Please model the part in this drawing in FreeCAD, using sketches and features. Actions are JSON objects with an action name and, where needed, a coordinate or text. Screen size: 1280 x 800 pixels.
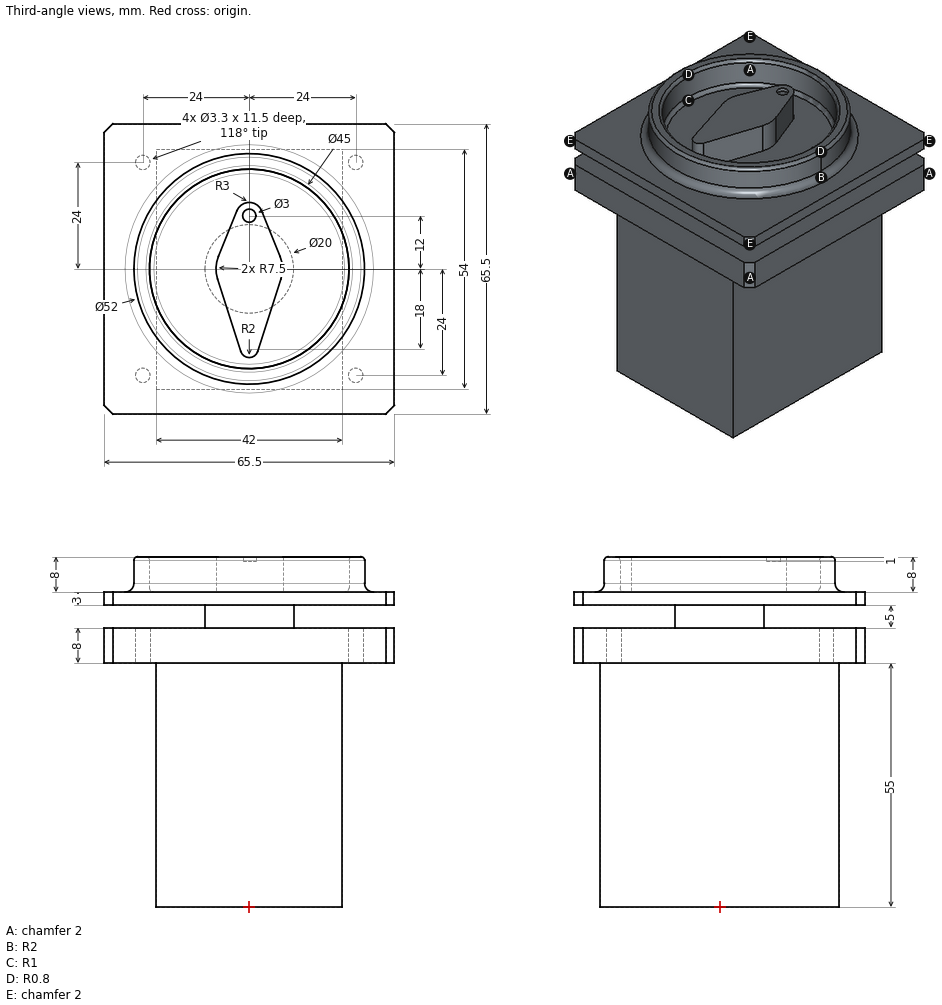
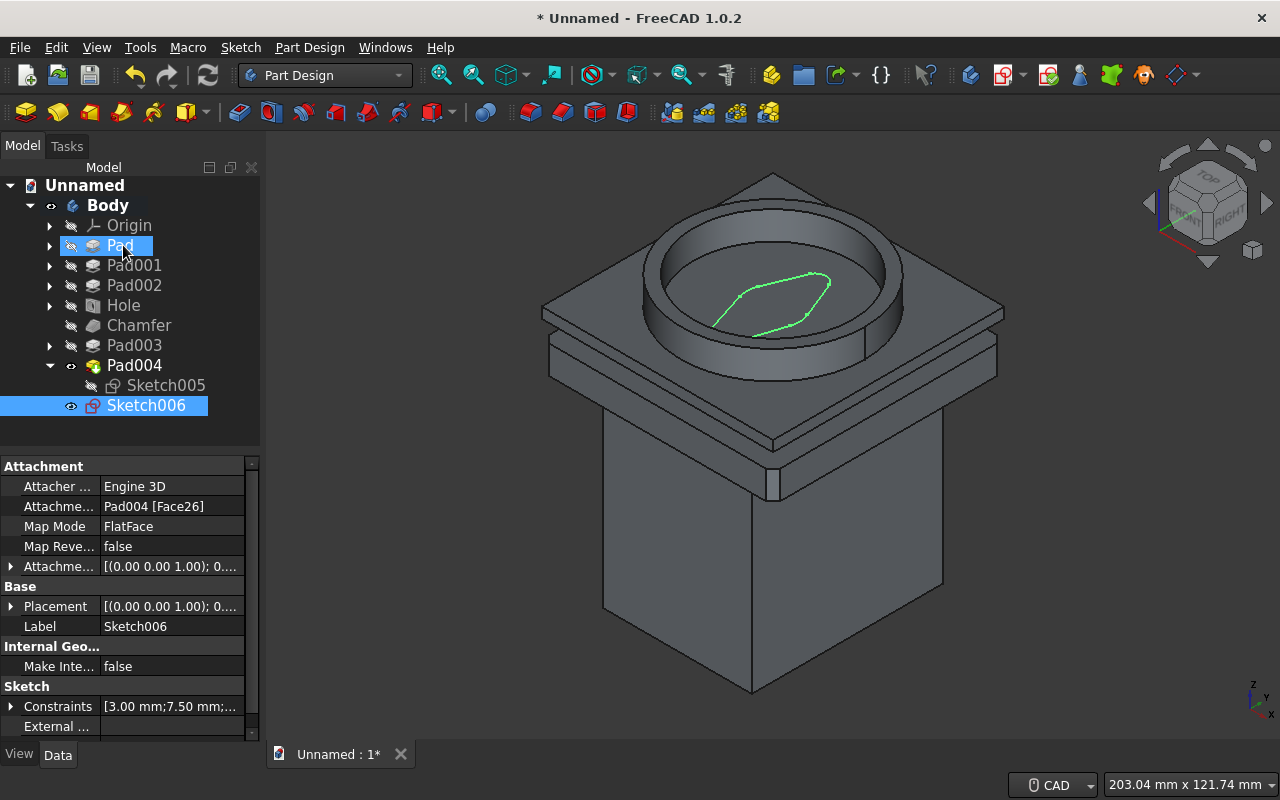
{"action": "left_click", "coordinate": [26, 112]}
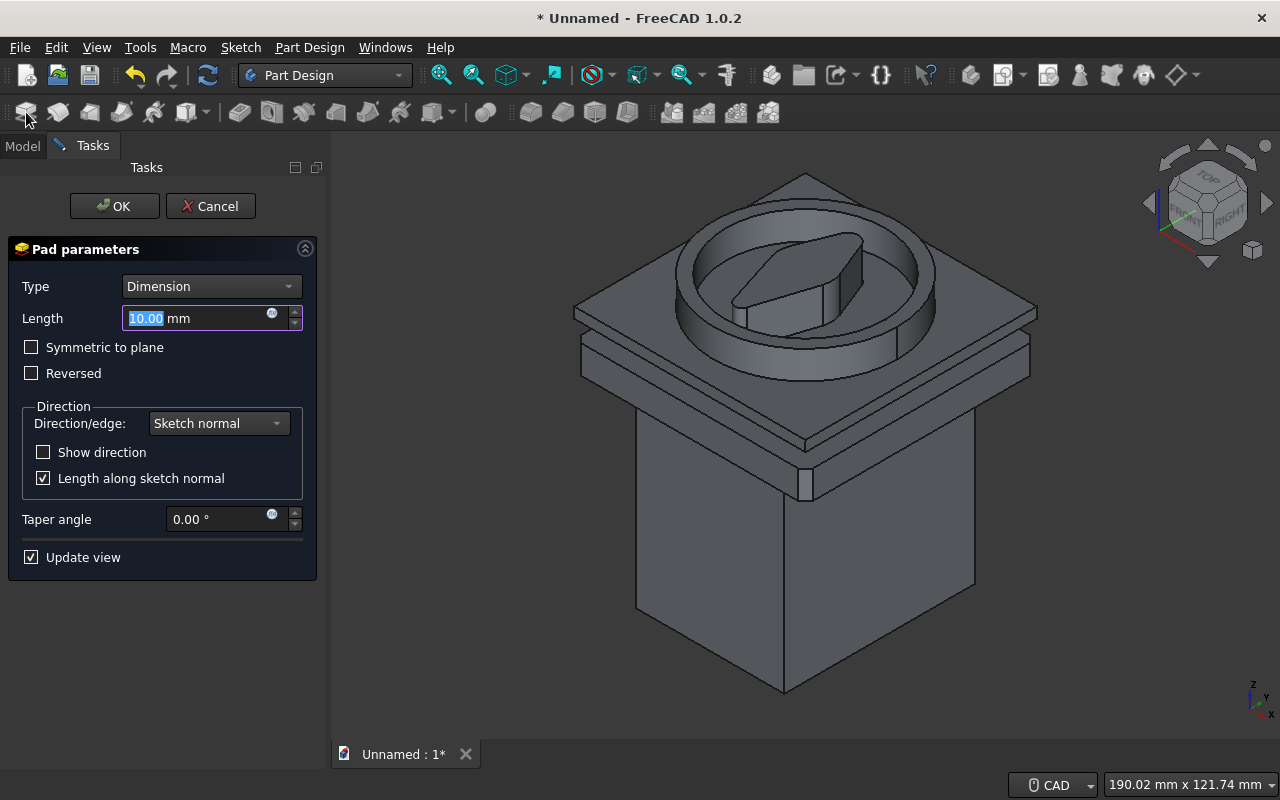
{"action": "type", "text": "8"}
{"action": "key", "text": "Tab"}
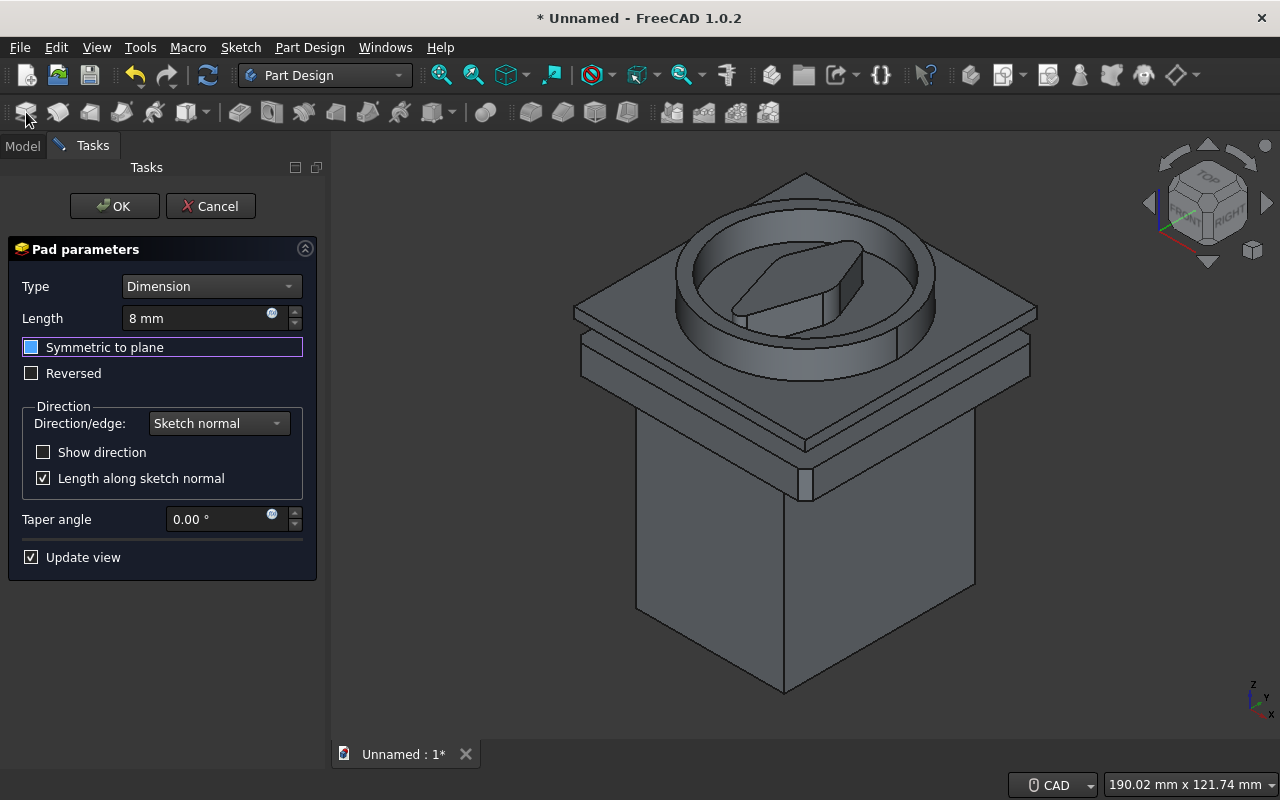
{"action": "left_click", "coordinate": [115, 206]}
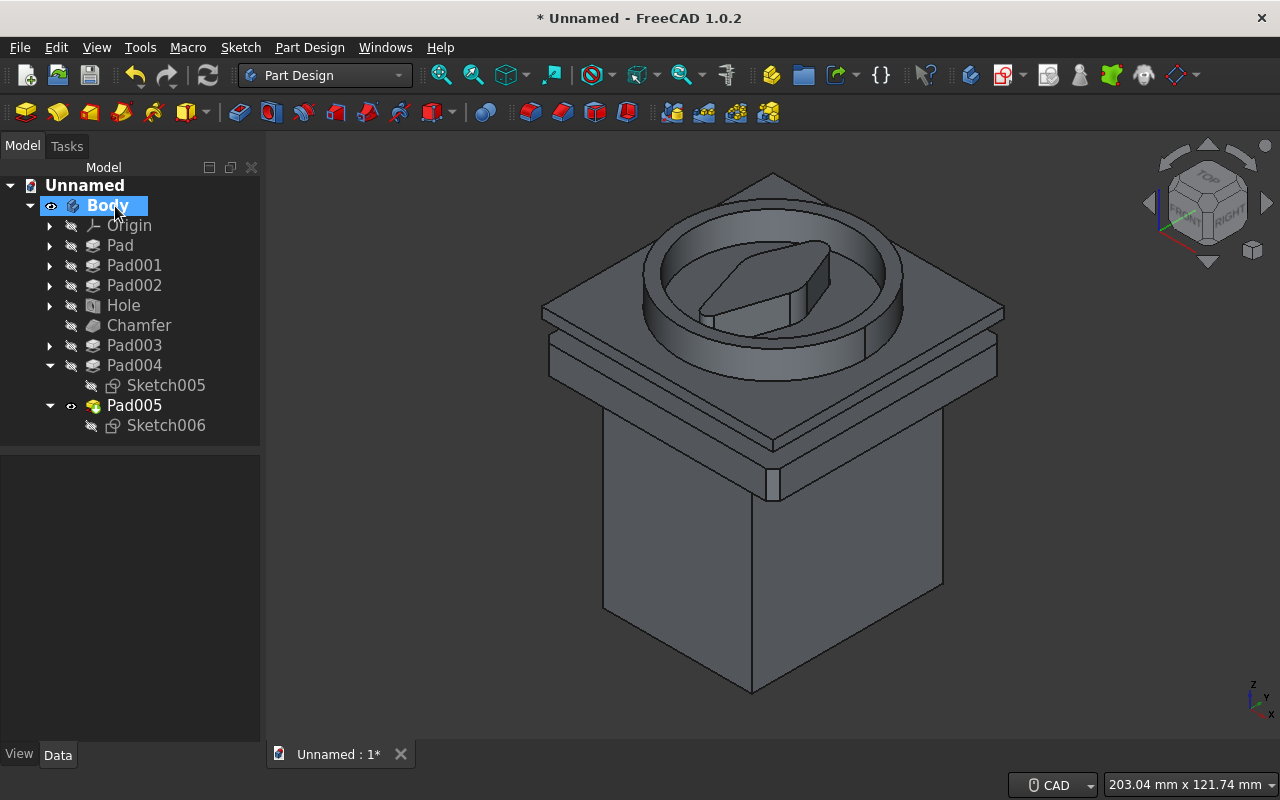
{"action": "key", "text": "2"}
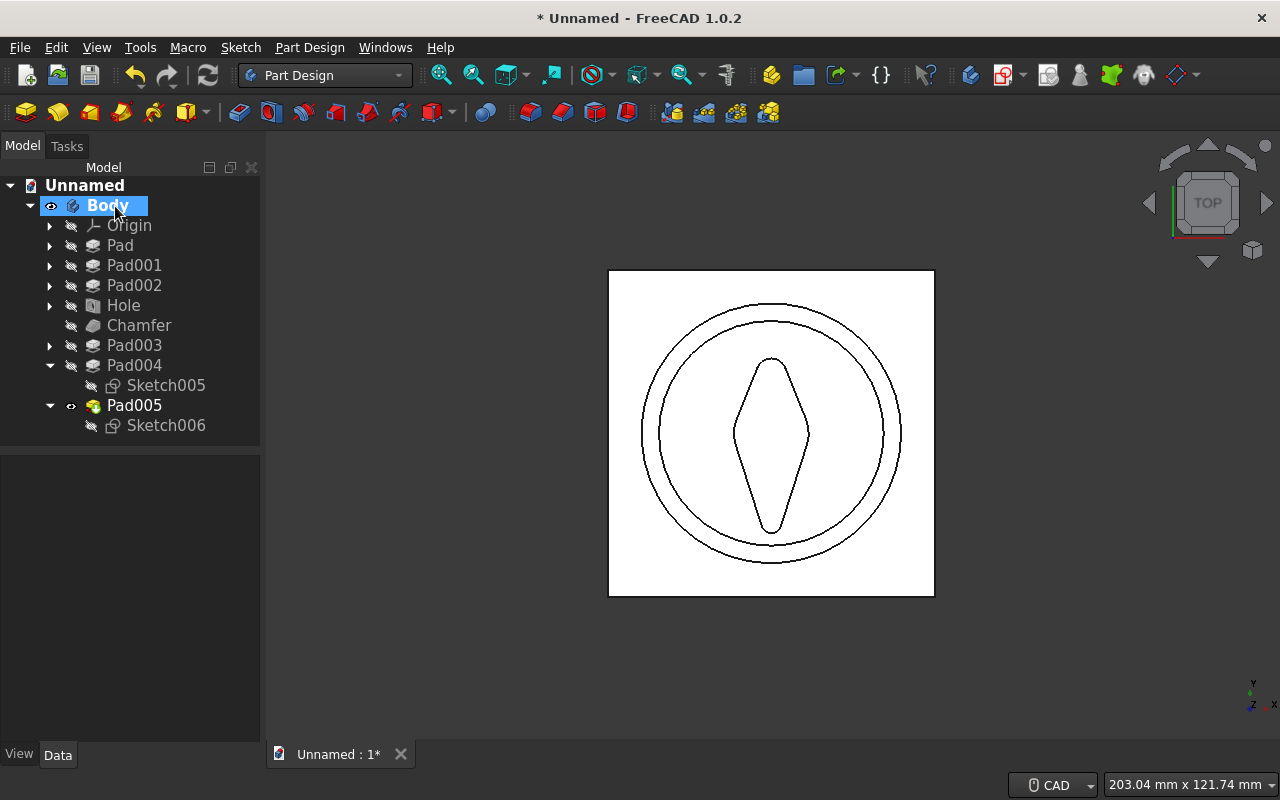
{"action": "key", "text": "0"}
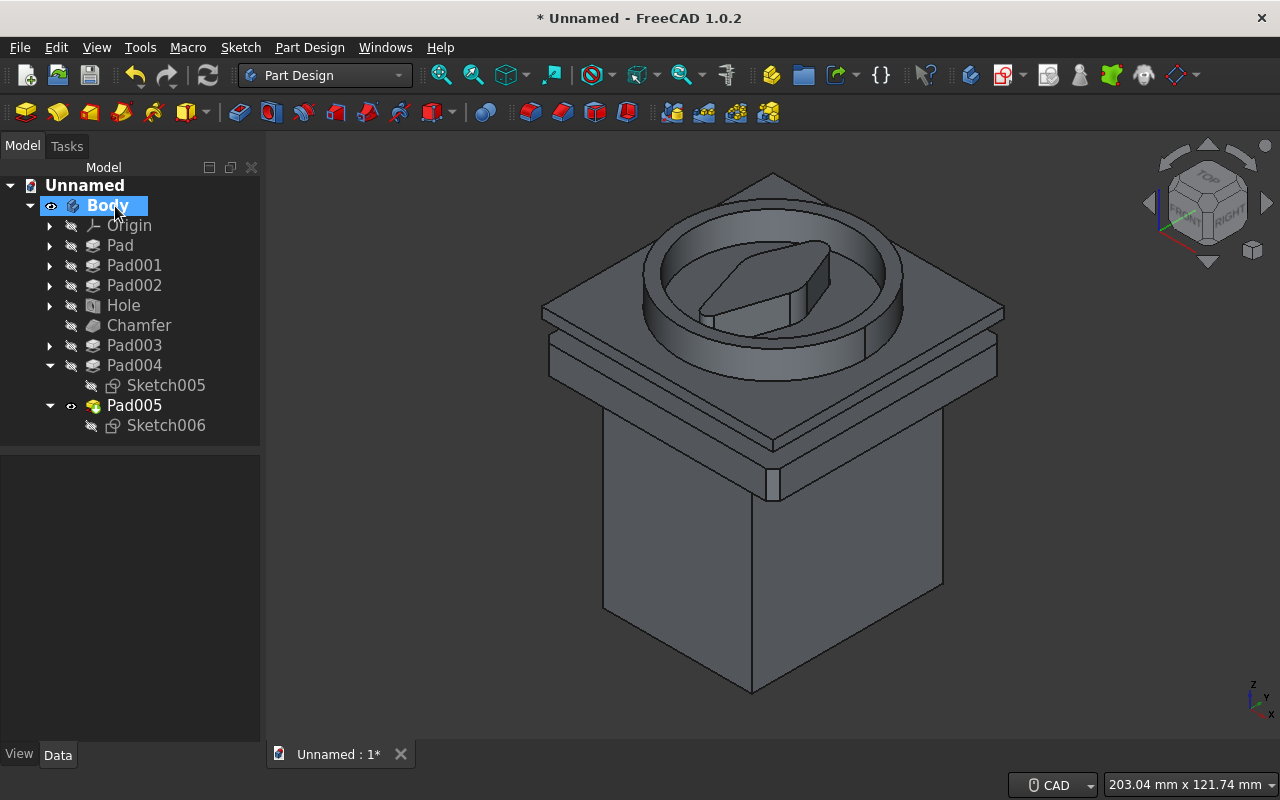
{"action": "key", "text": "1"}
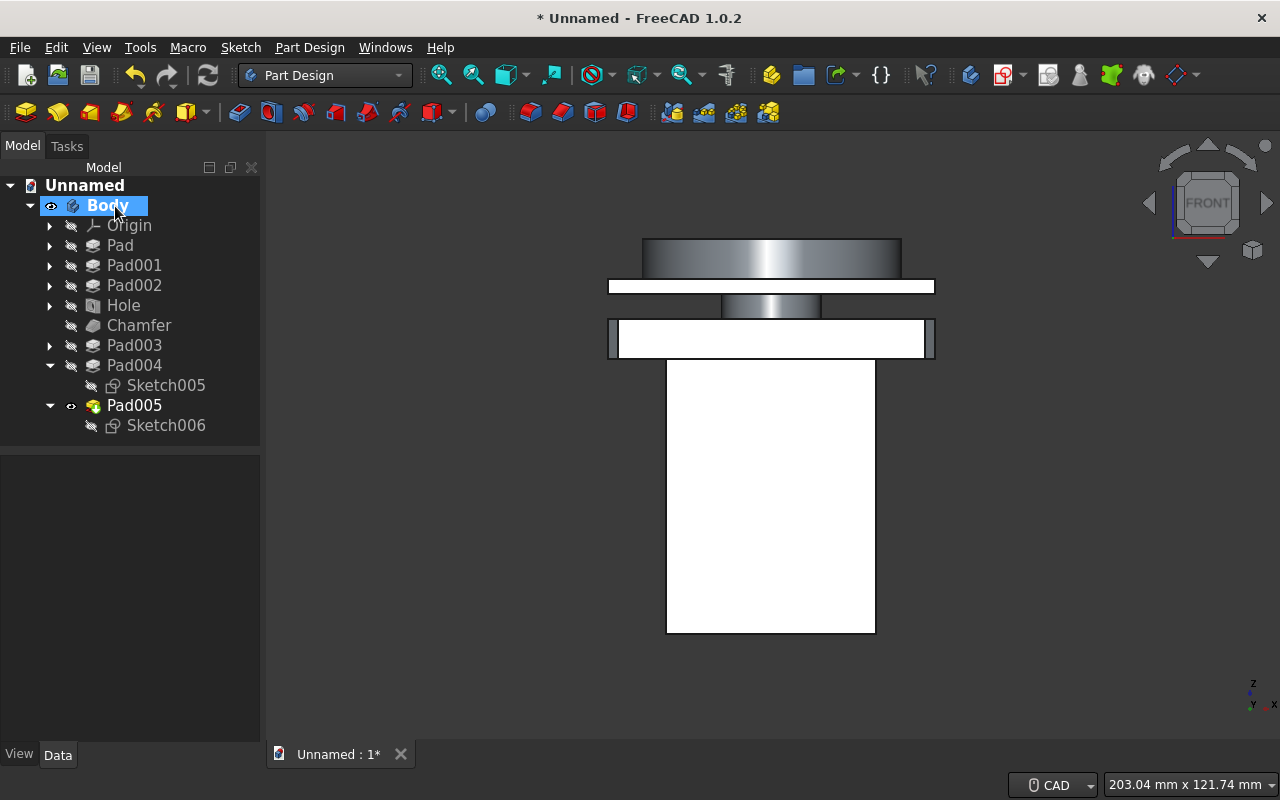
{"action": "key", "text": "3"}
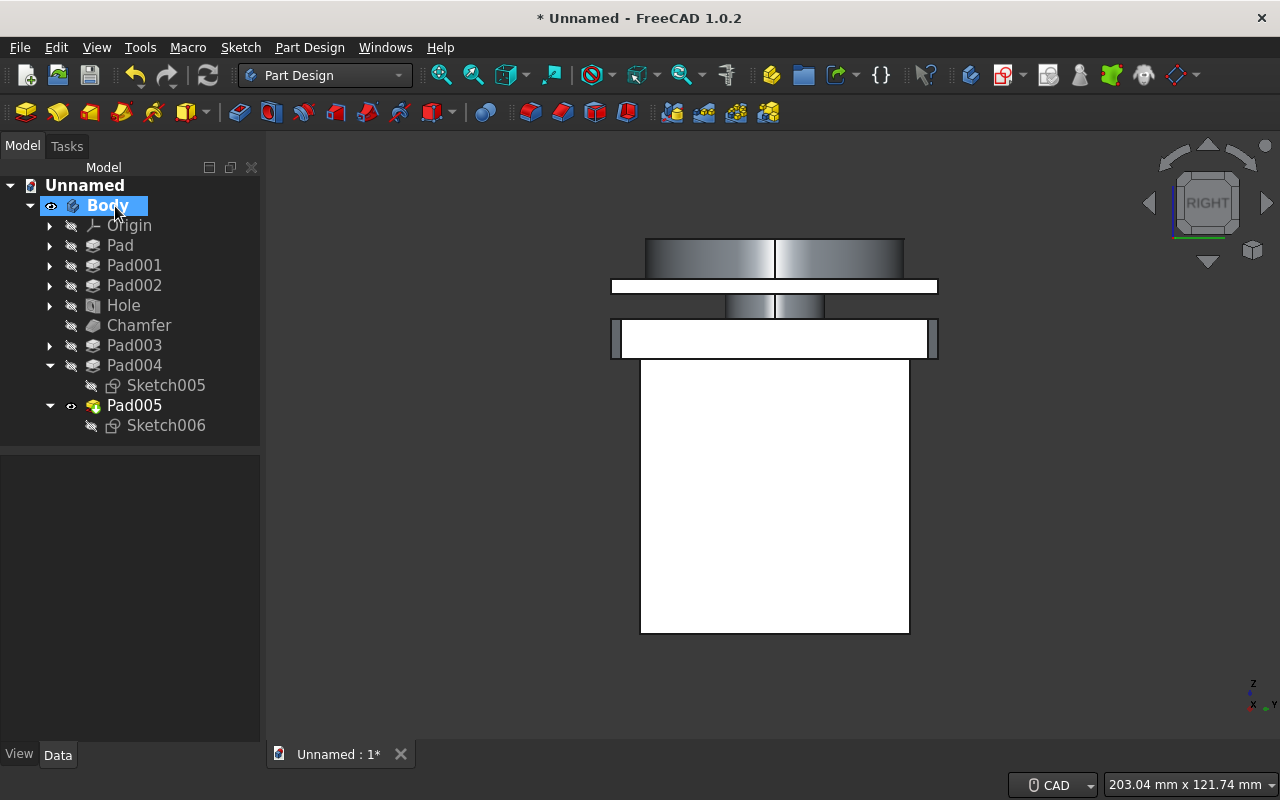
{"action": "key", "text": "5"}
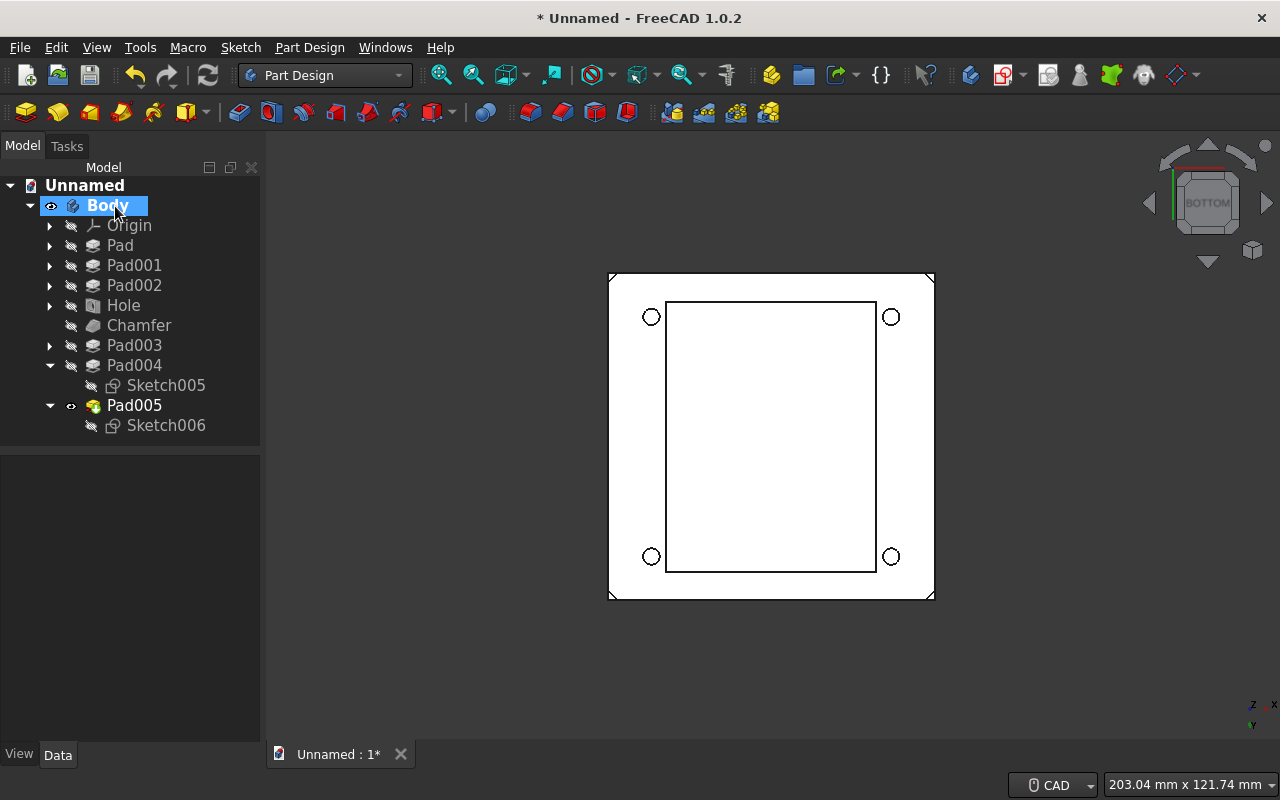
{"action": "key", "text": "4"}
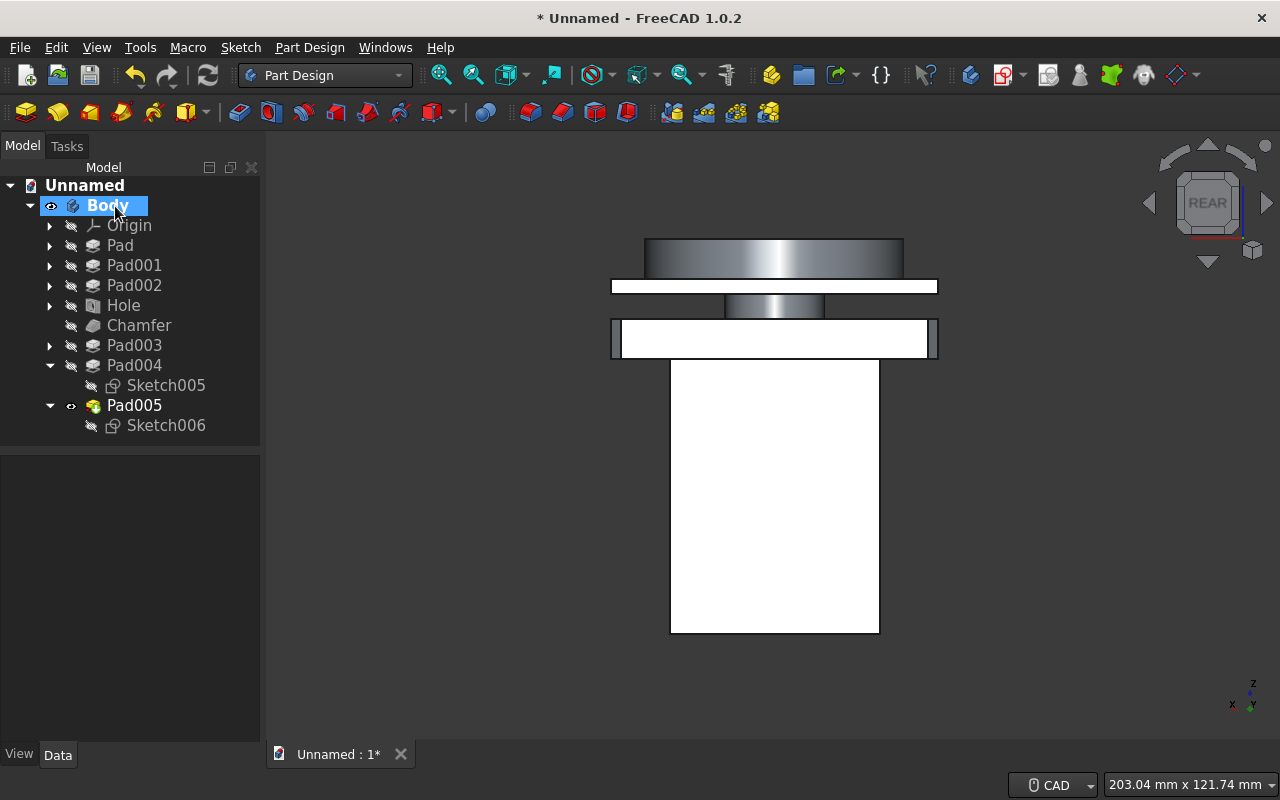
{"action": "key", "text": "6"}